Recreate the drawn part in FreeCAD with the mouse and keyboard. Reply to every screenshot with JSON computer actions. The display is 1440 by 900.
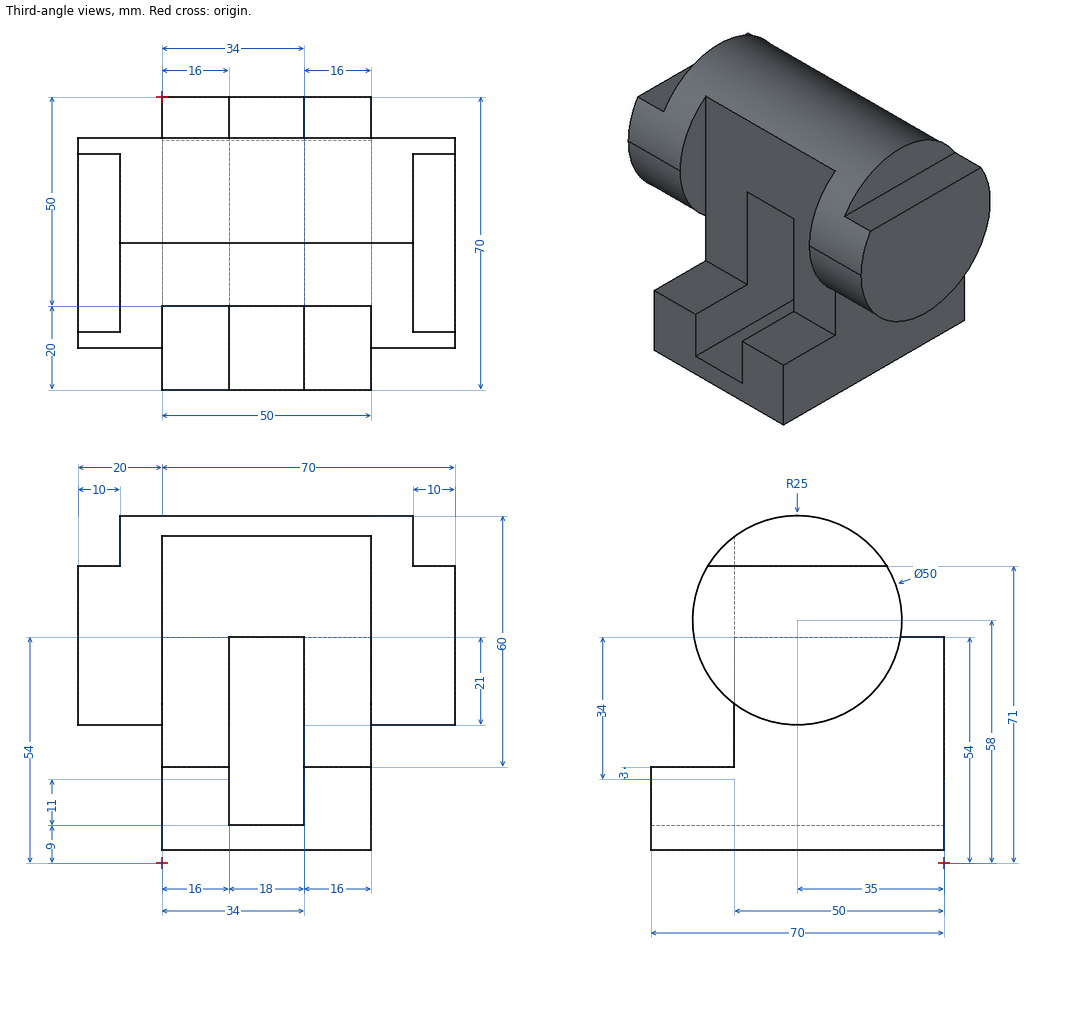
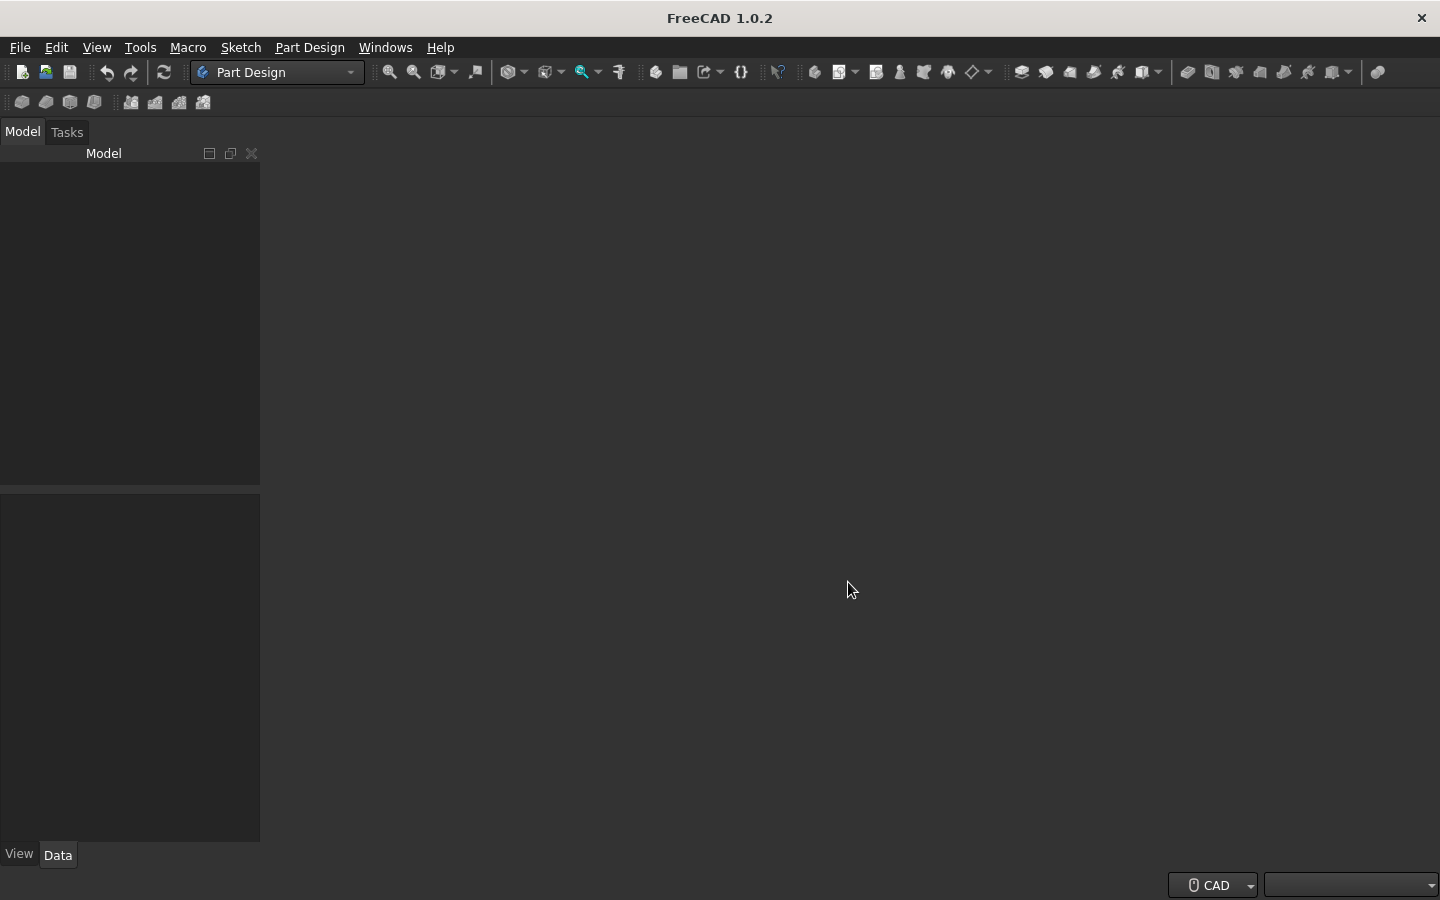
{"action": "left_click", "coordinate": [22, 72]}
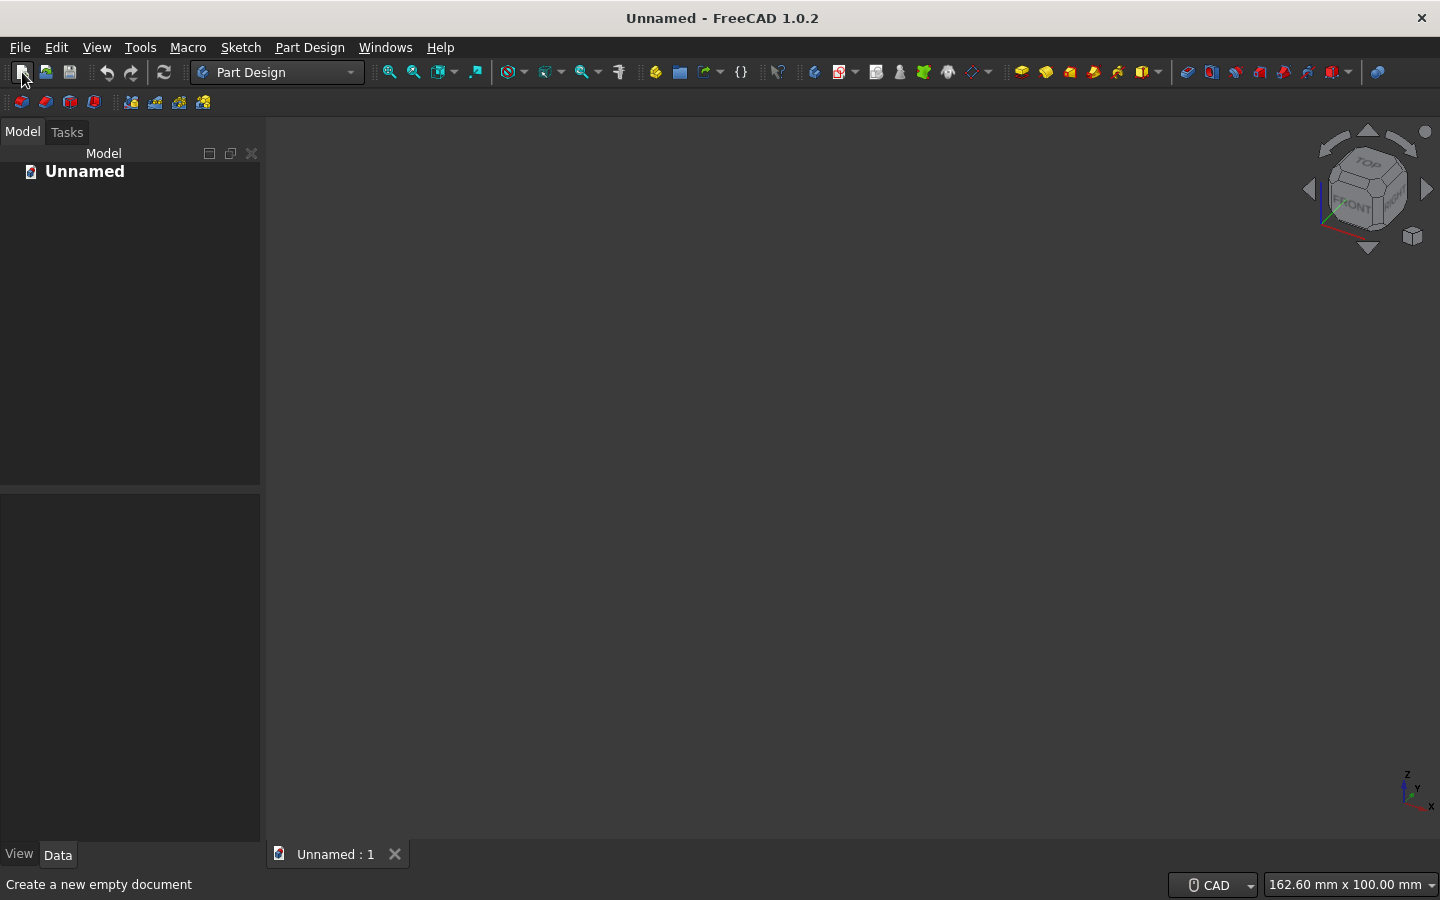
{"action": "left_click", "coordinate": [840, 72]}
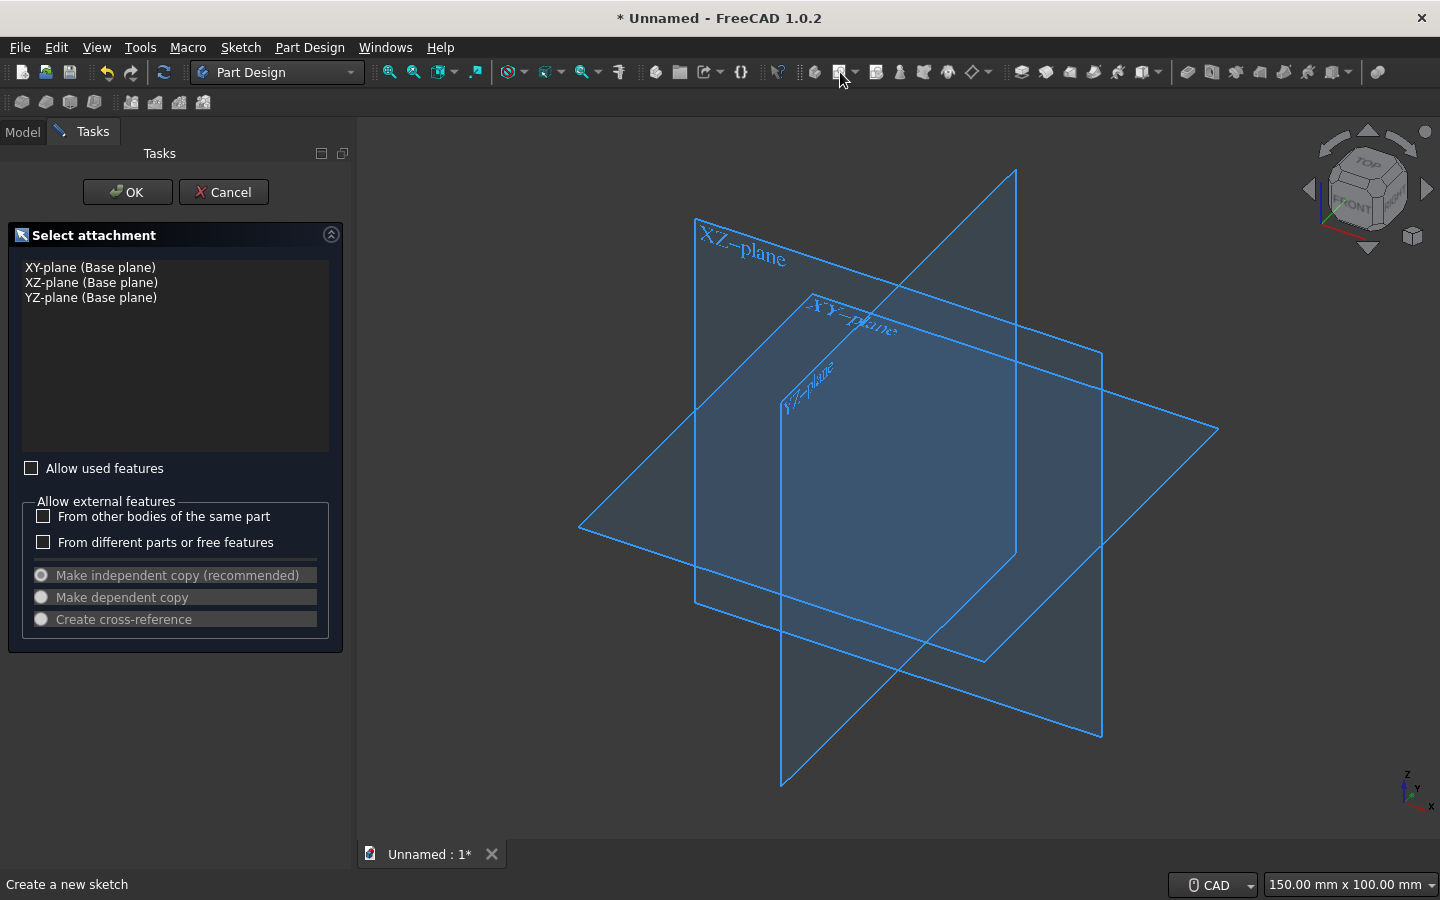
{"action": "left_click", "coordinate": [82, 268]}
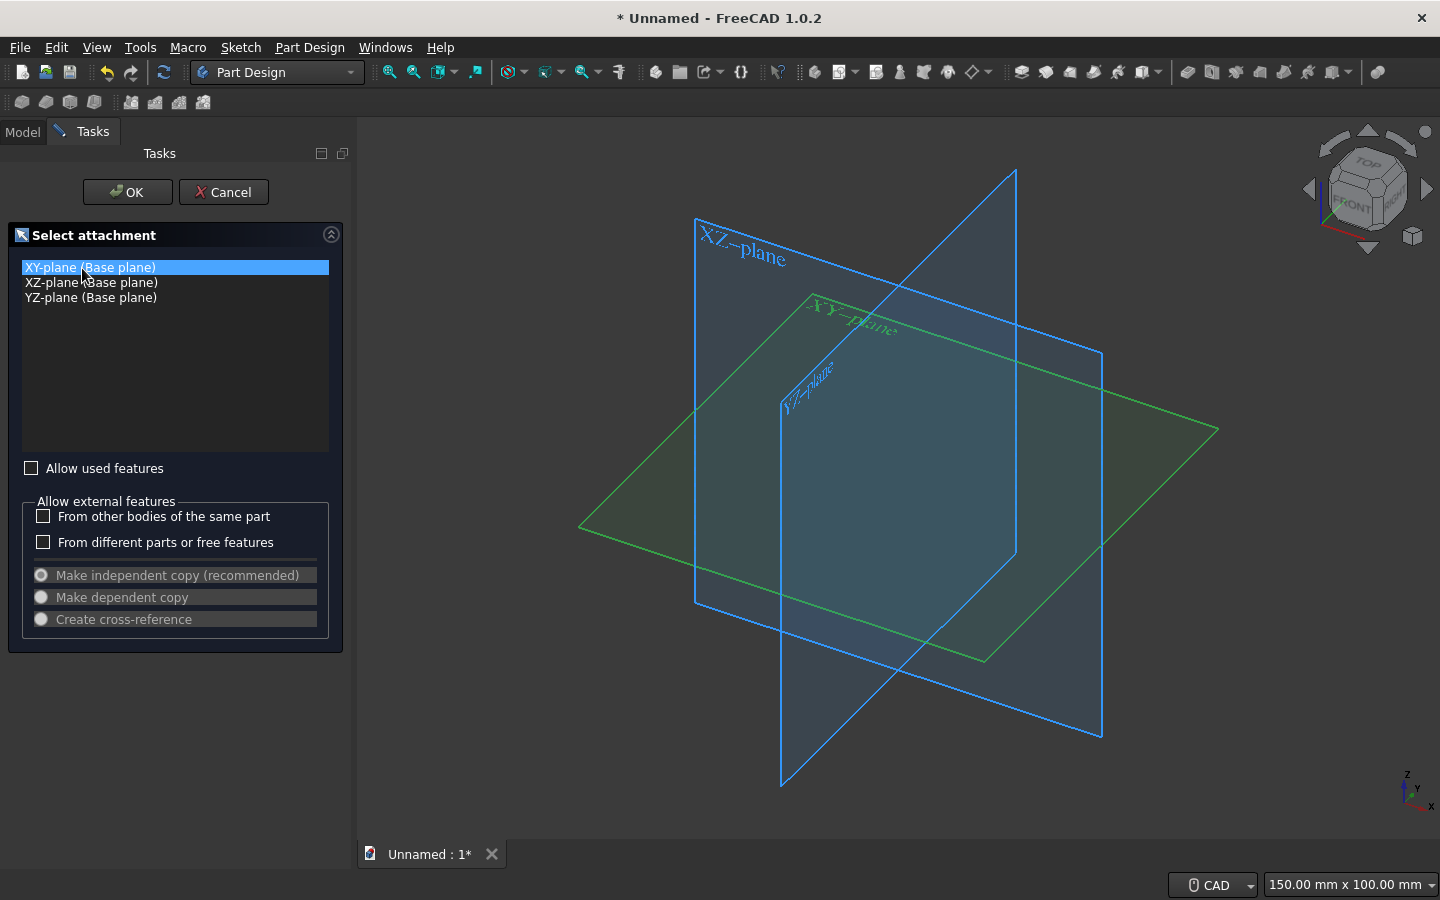
{"action": "left_click", "coordinate": [128, 192]}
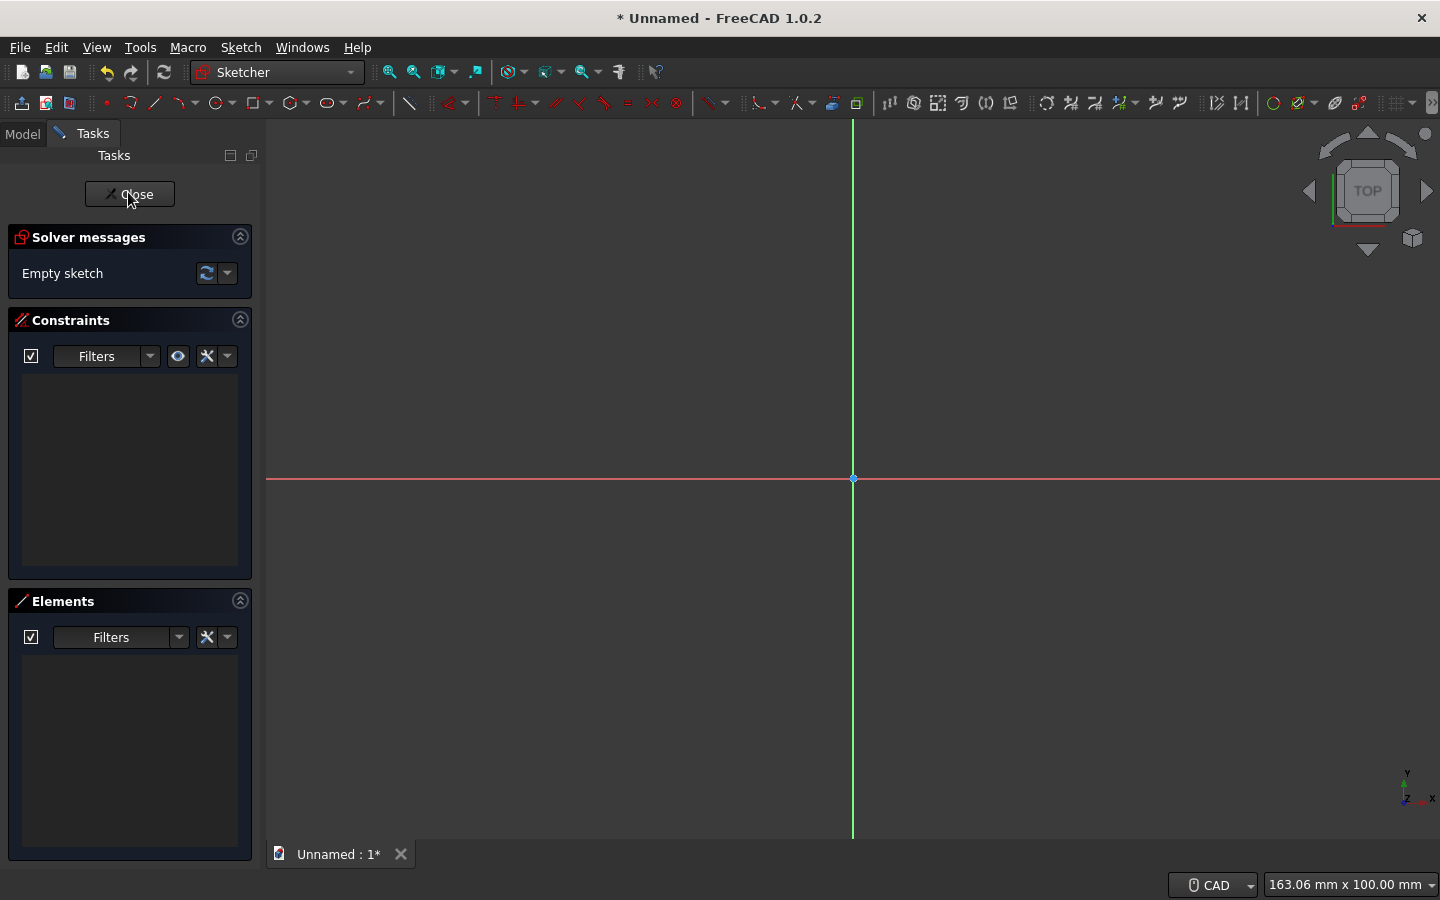
{"action": "scroll", "coordinate": [294, 147], "scroll_direction": "down", "scroll_amount": 2}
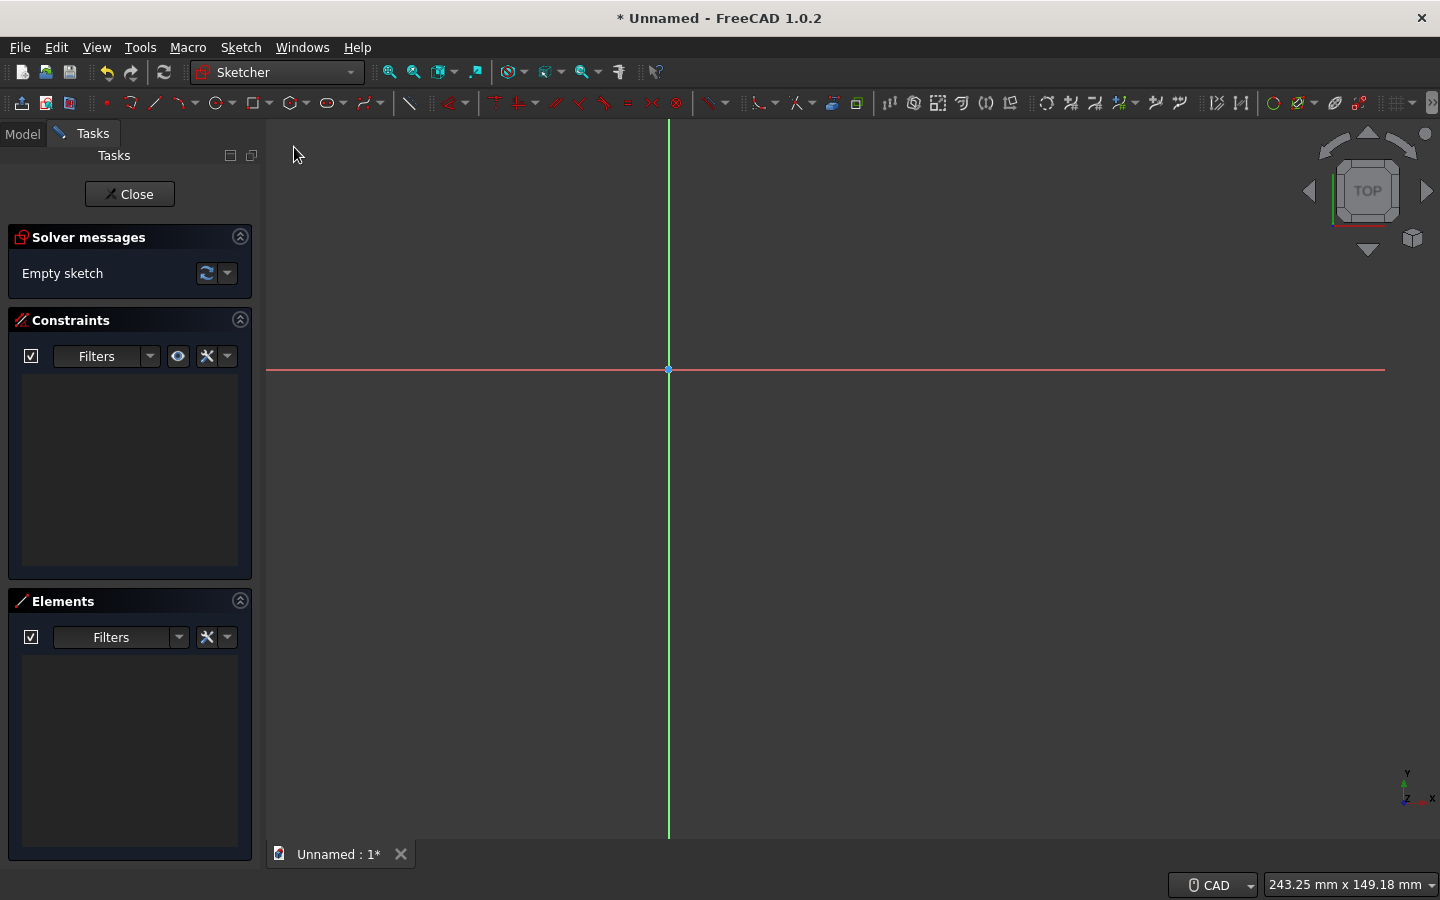
{"action": "scroll", "coordinate": [799, 659], "scroll_direction": "up", "scroll_amount": 2}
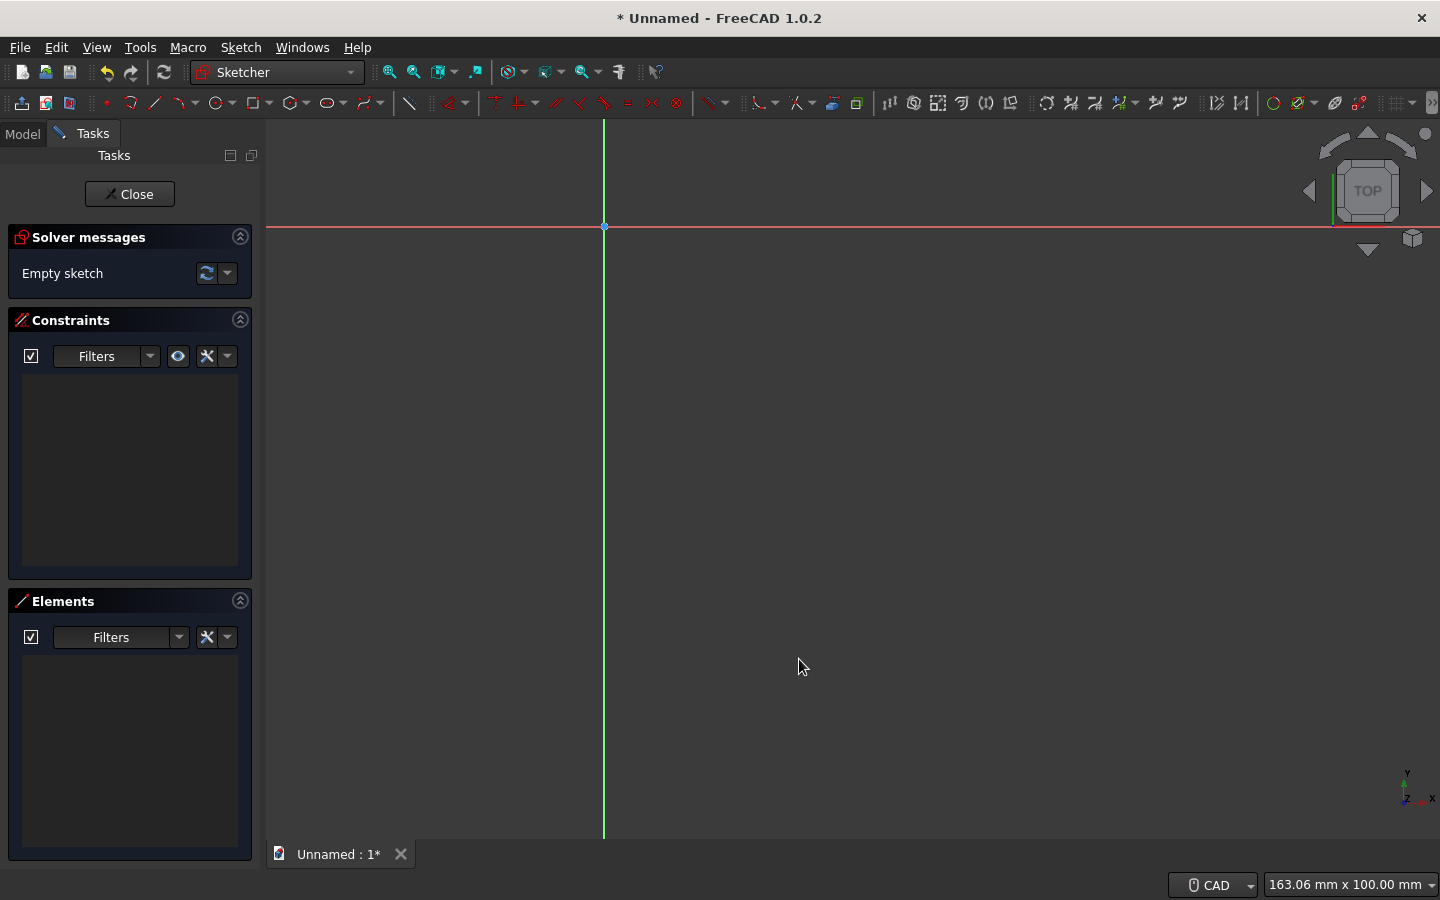
{"action": "key", "text": "g r"}